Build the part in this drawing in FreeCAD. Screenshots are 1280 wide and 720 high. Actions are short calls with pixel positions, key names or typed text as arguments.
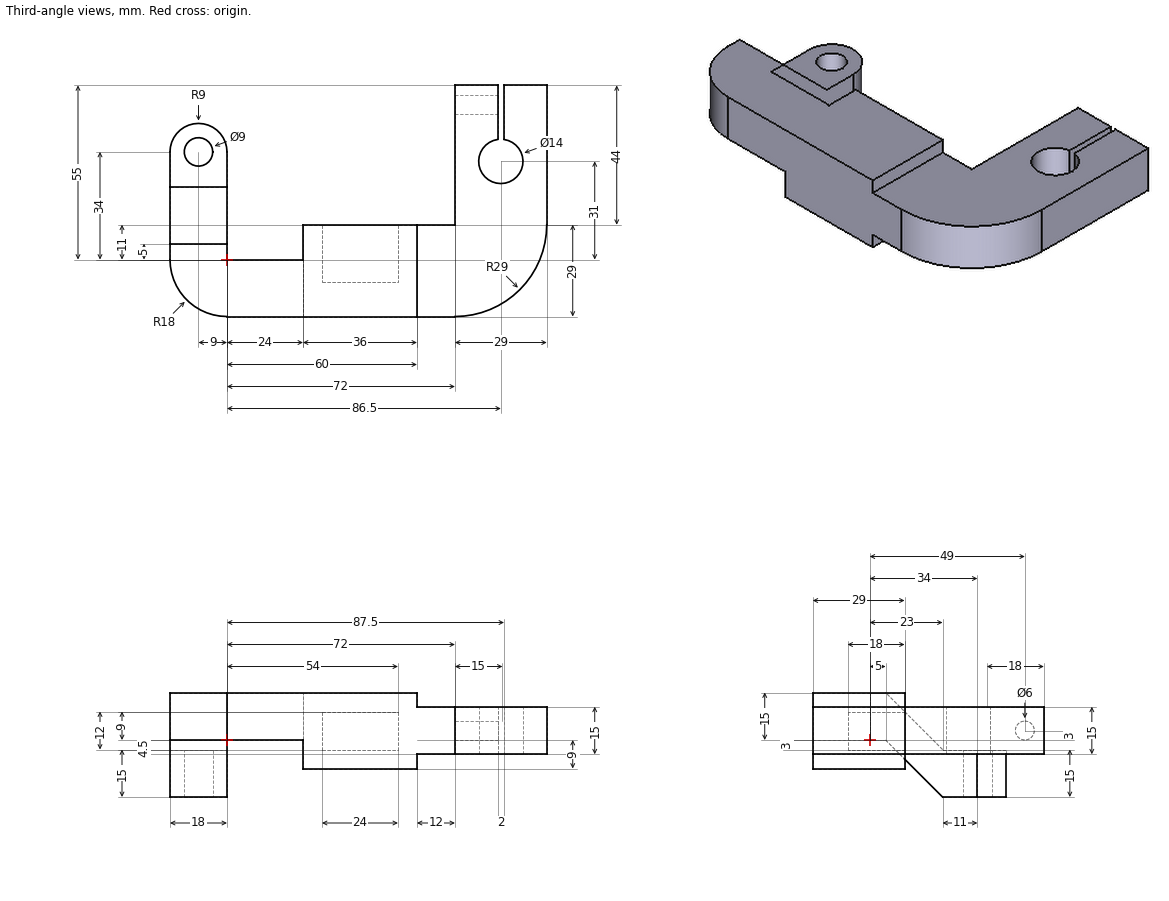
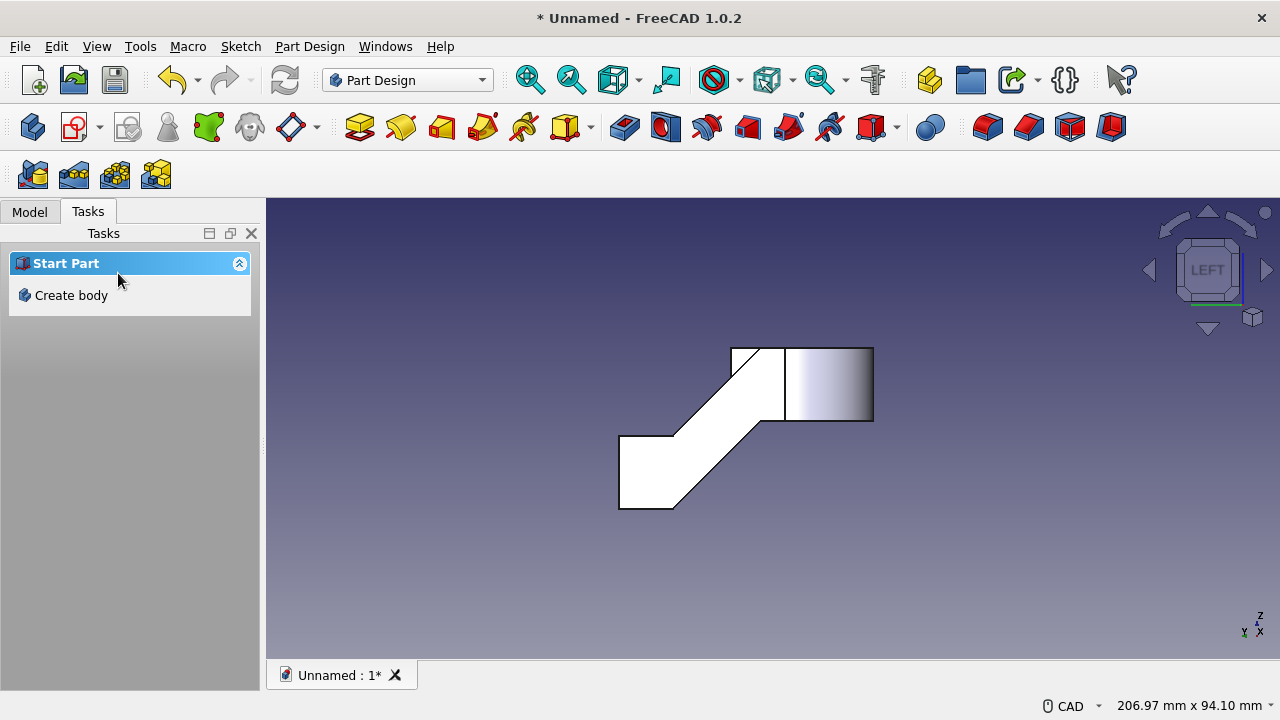
click(531, 80)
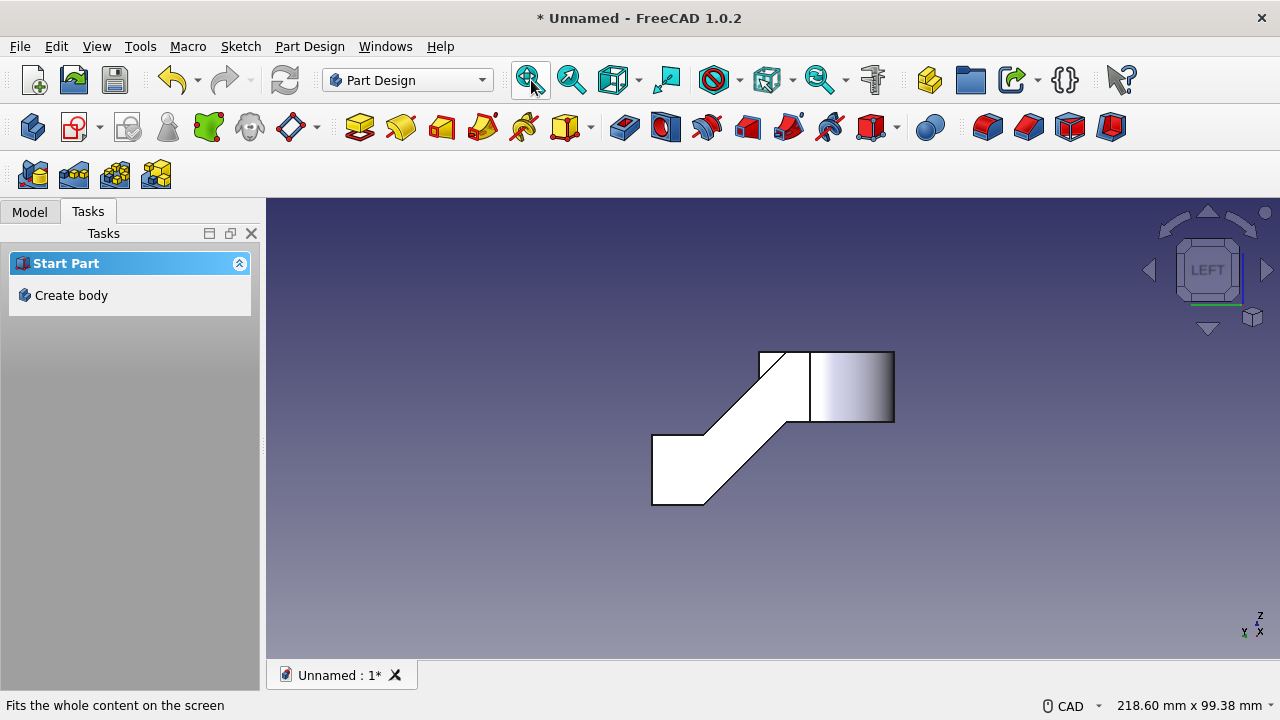
key(0)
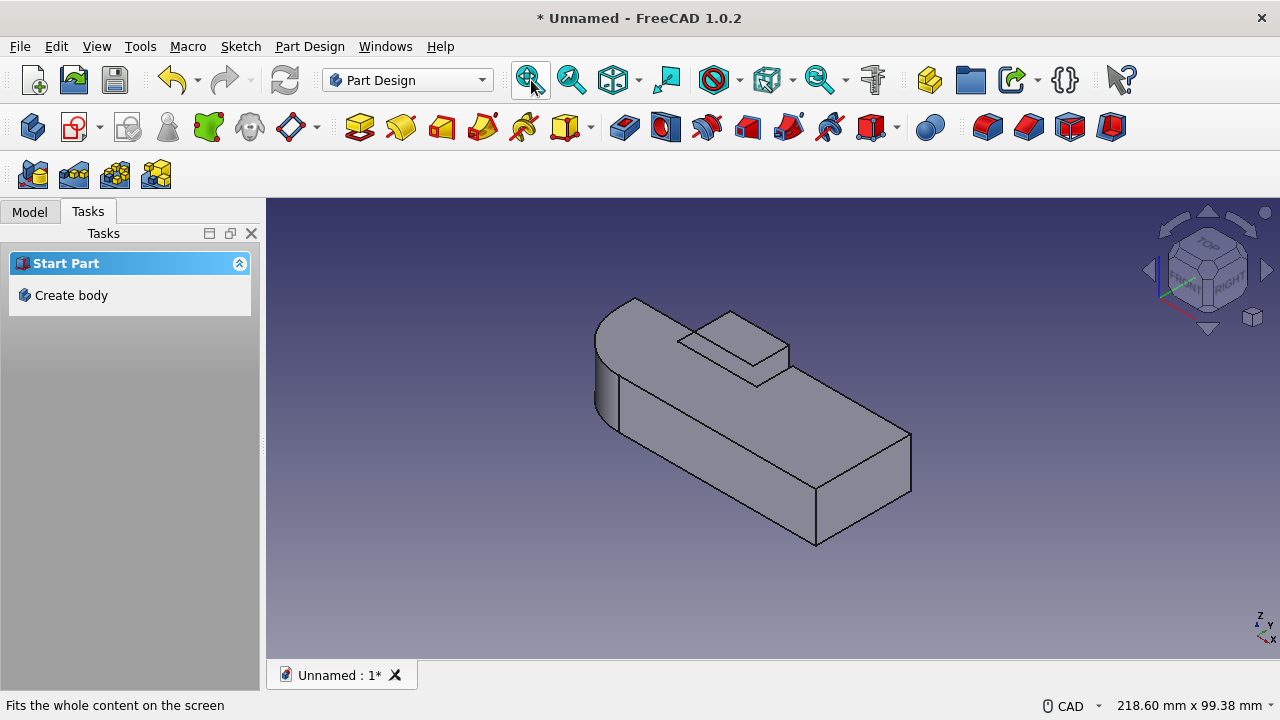
click(750, 342)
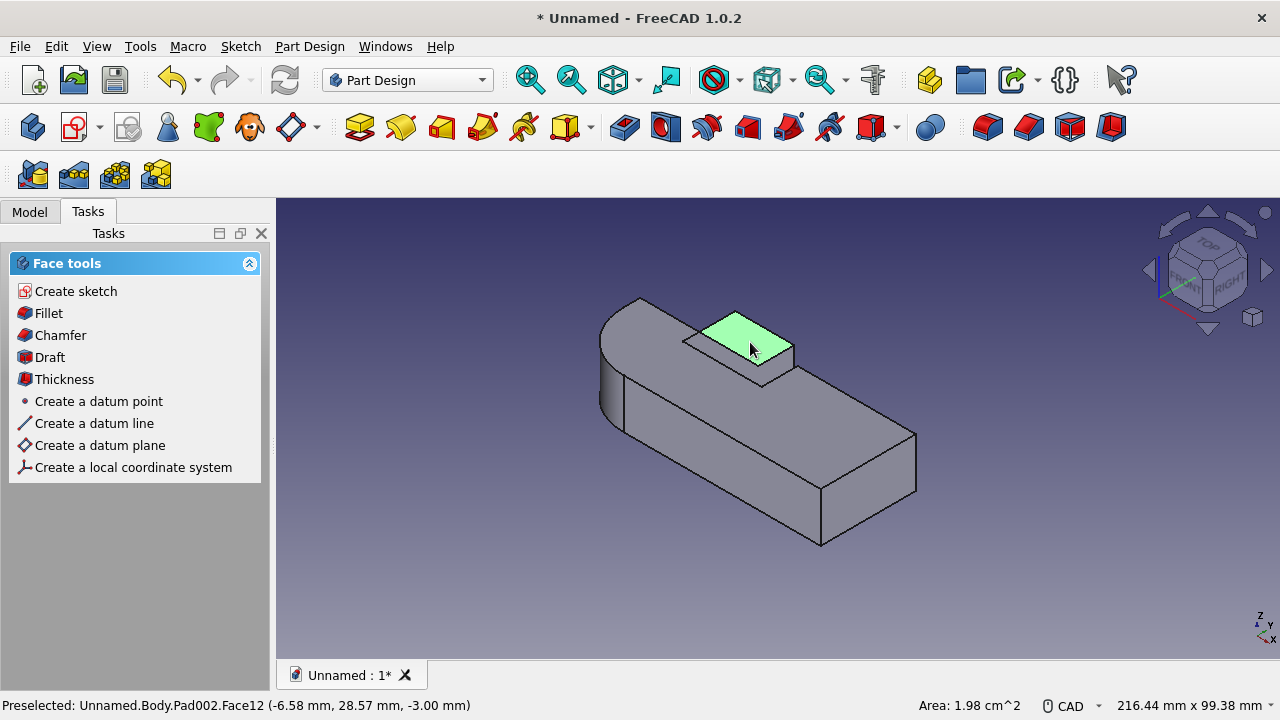
click(74, 128)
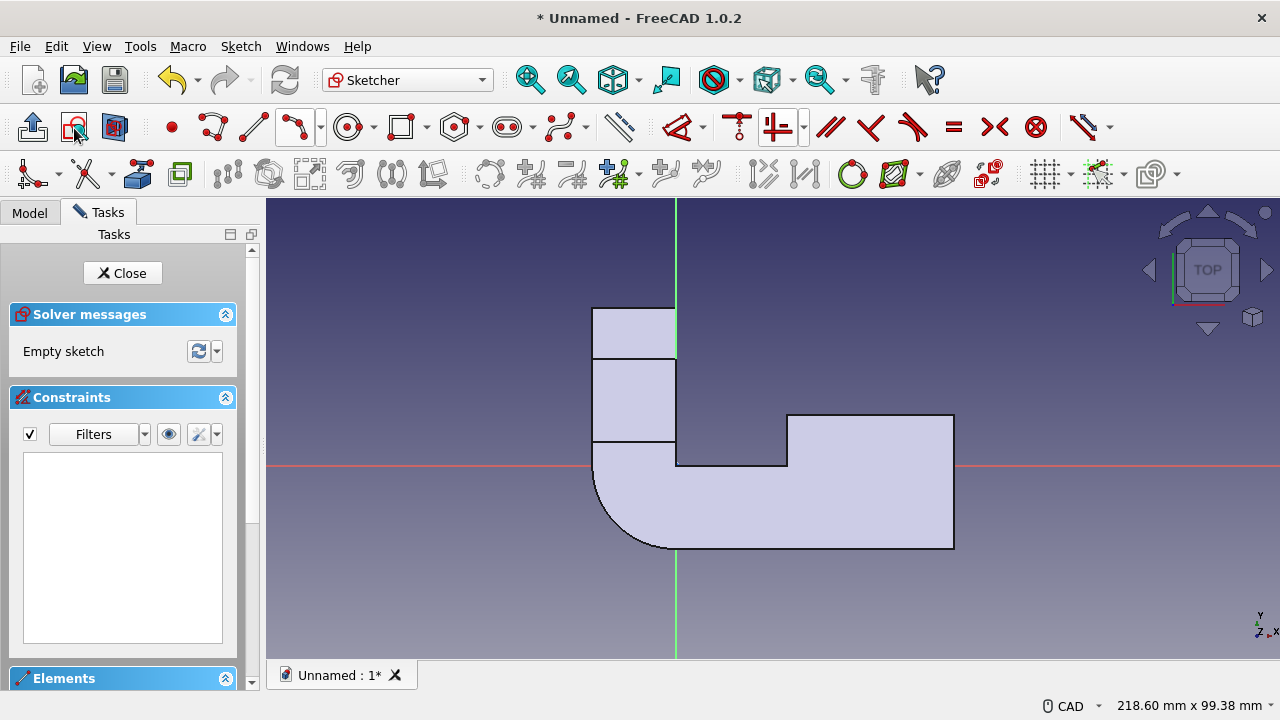
scroll(490, 239, up, 2)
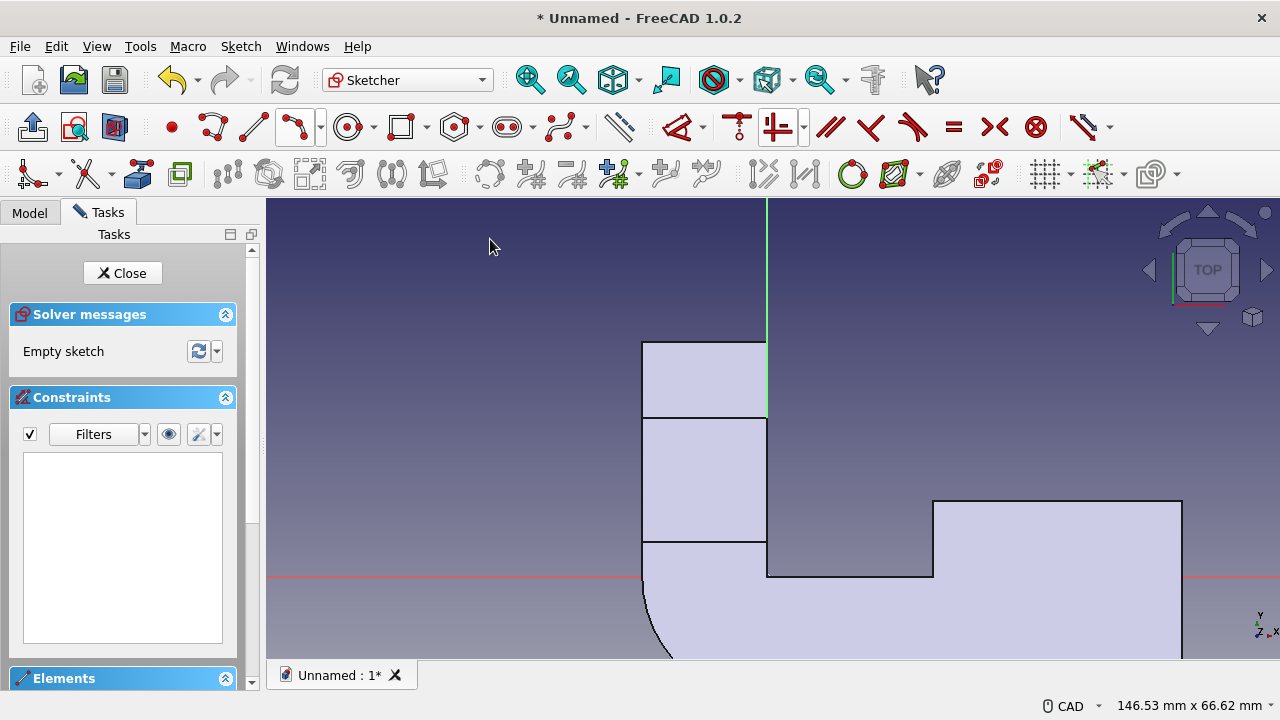
click(254, 128)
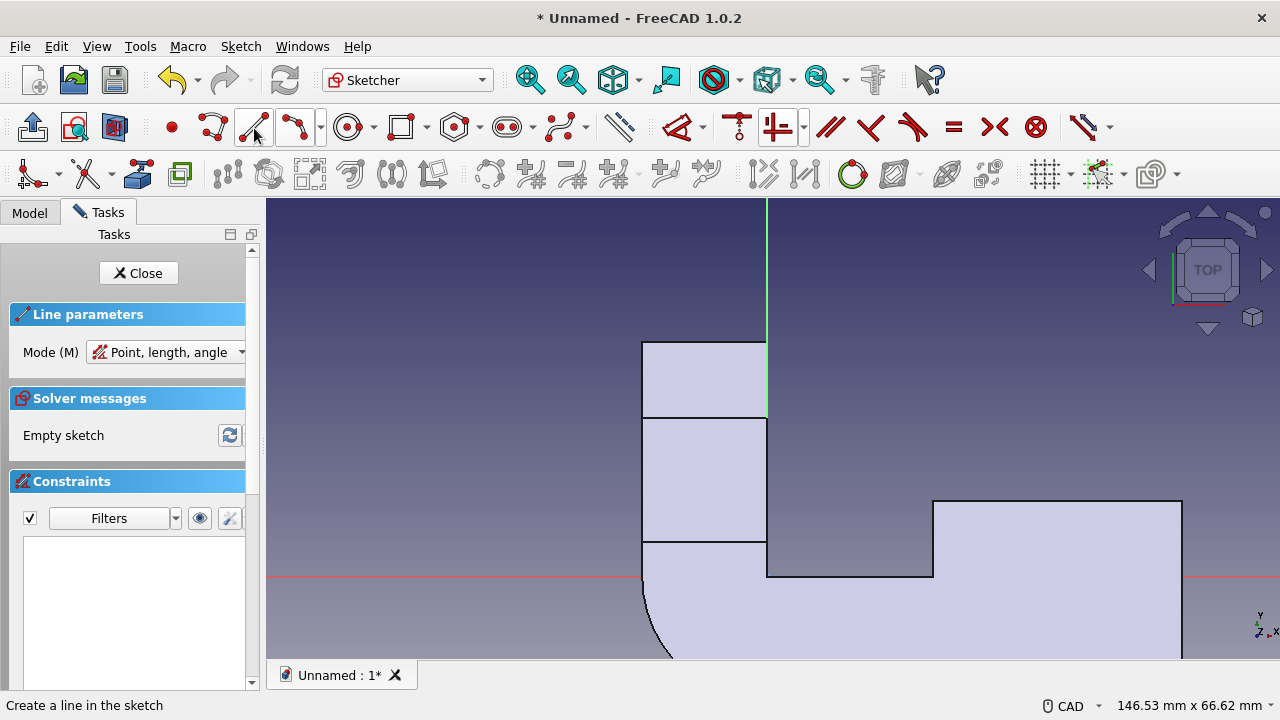
click(642, 342)
click(767, 342)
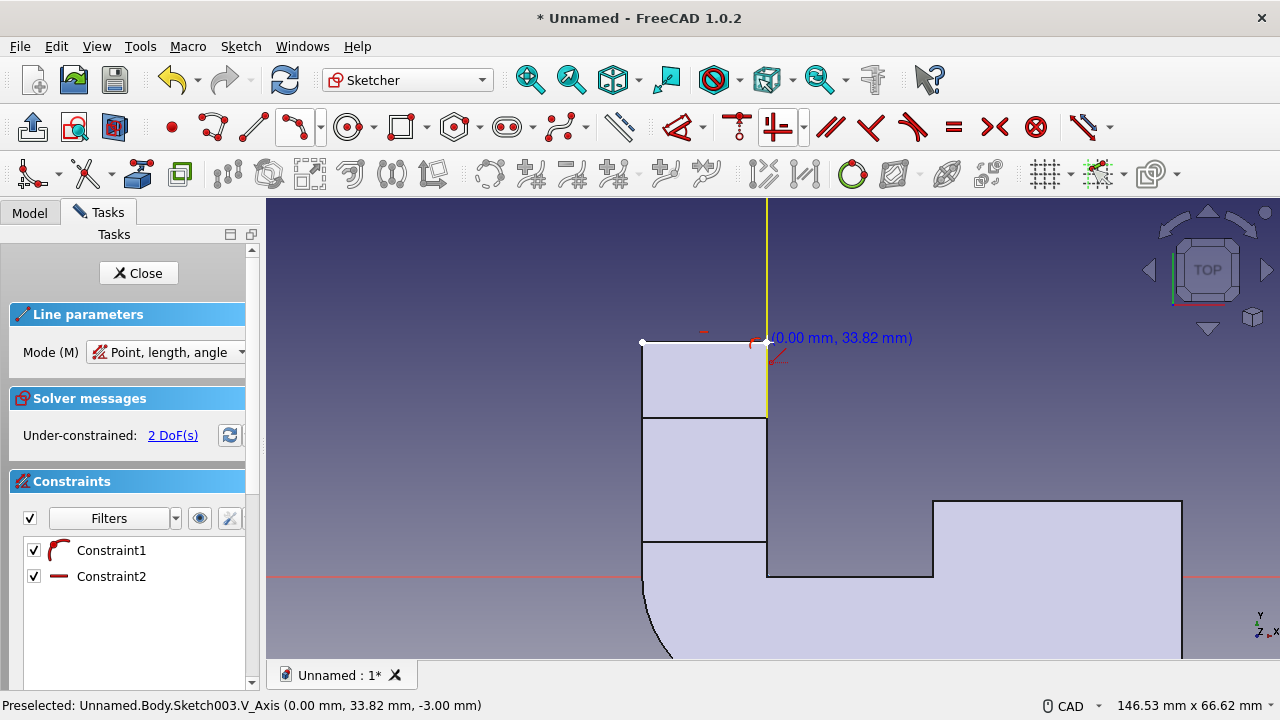
click(294, 128)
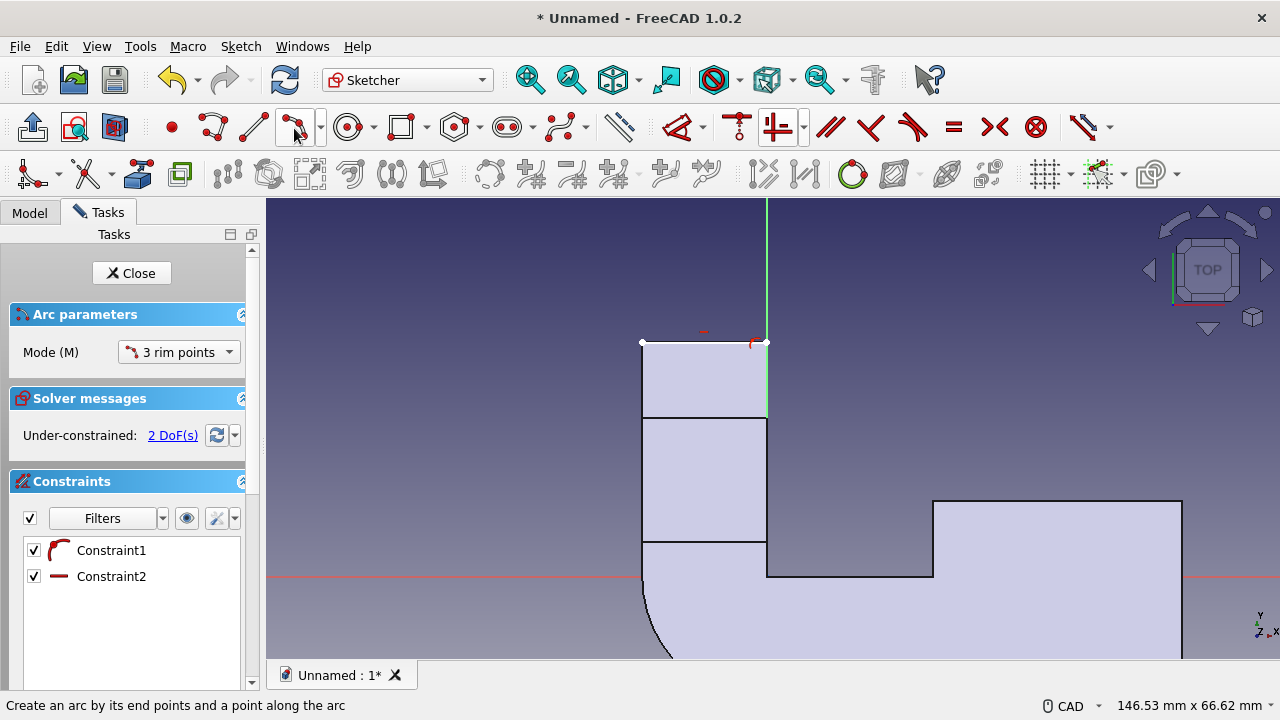
click(767, 343)
click(642, 343)
click(704, 279)
key(Escape)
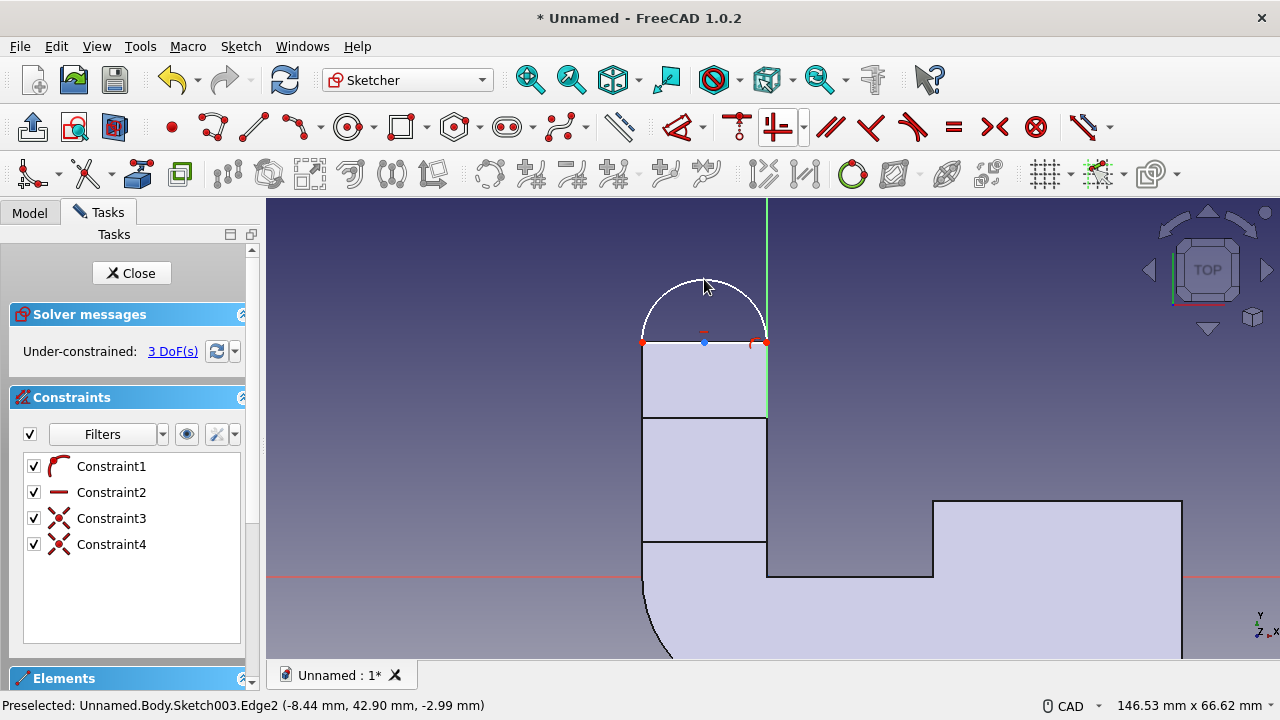
click(676, 128)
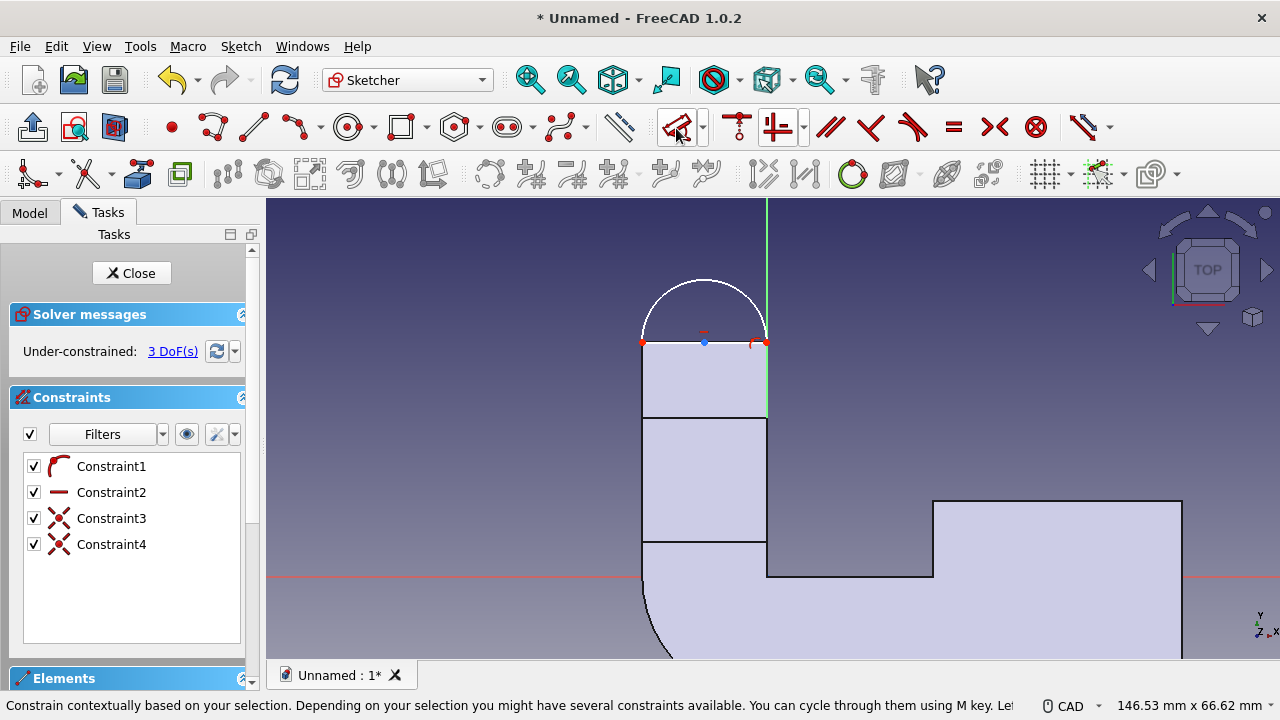
click(741, 292)
click(790, 302)